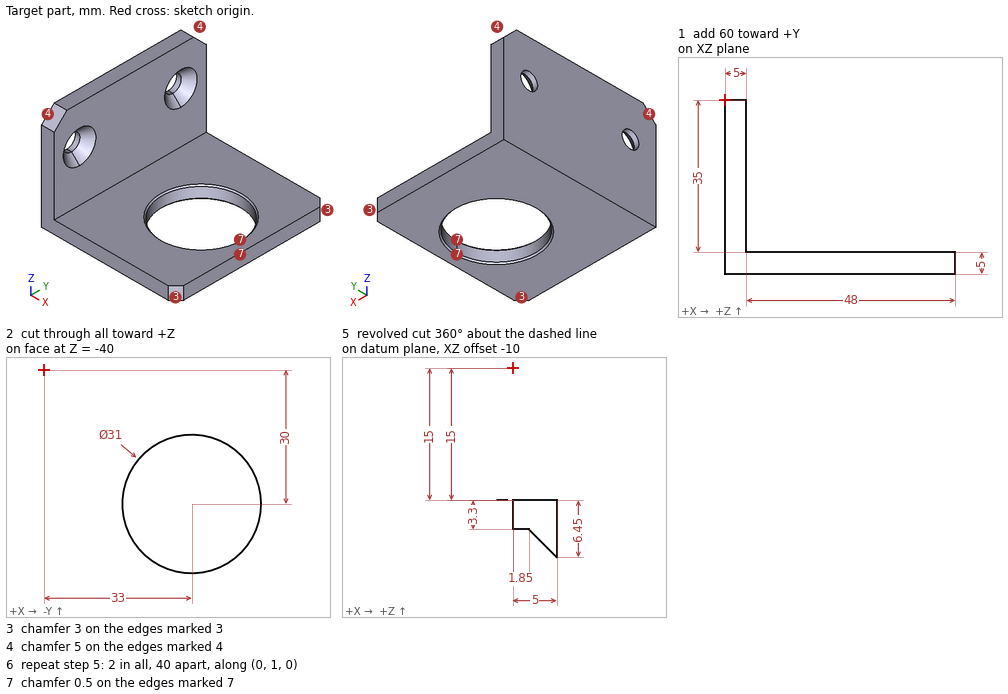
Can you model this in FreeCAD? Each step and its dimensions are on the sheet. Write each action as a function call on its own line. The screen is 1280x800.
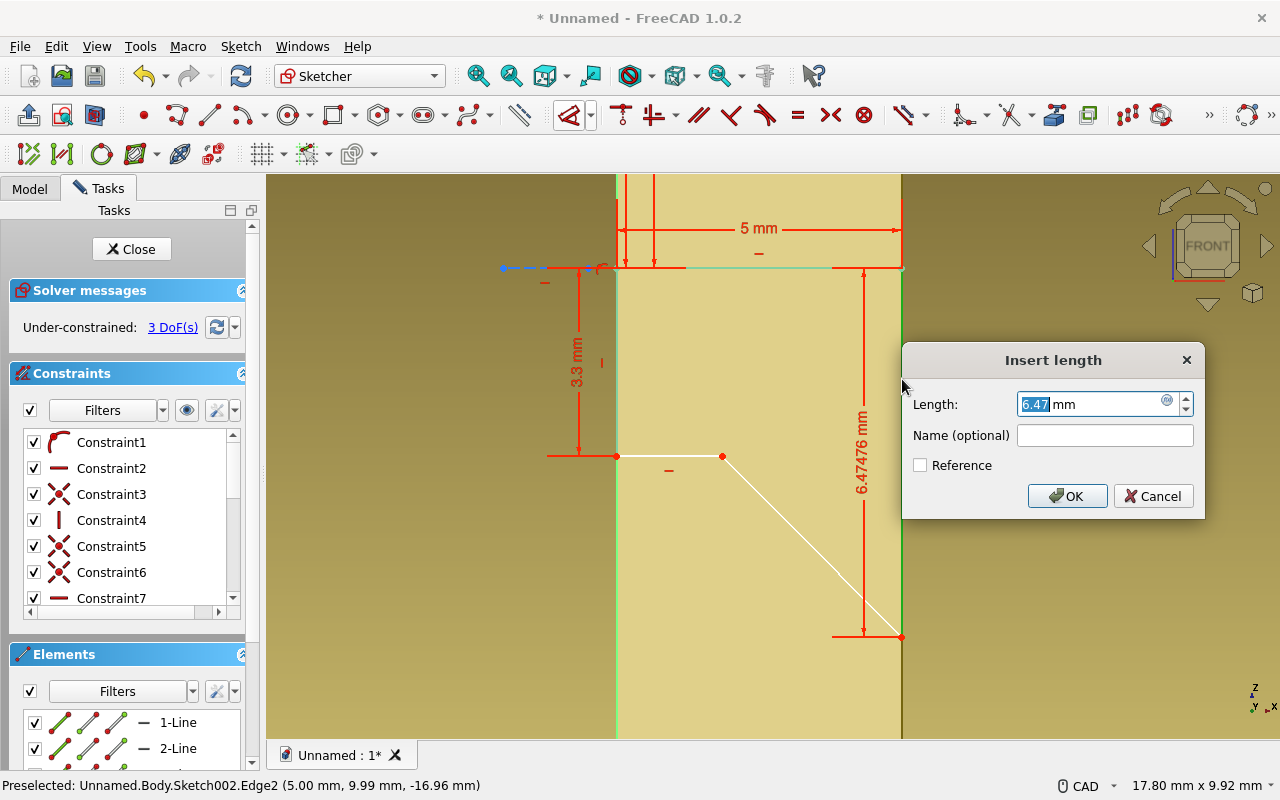
text(6.45)
key(Return)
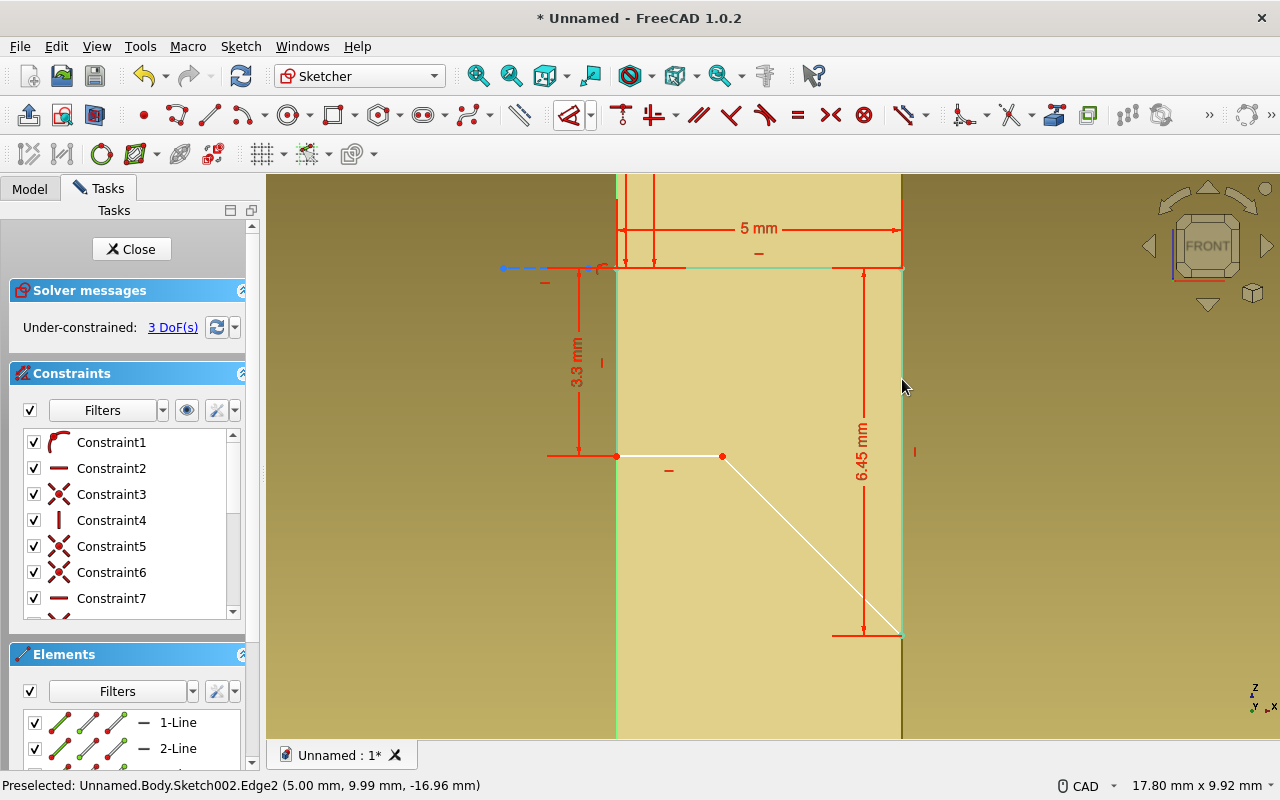
click(690, 456)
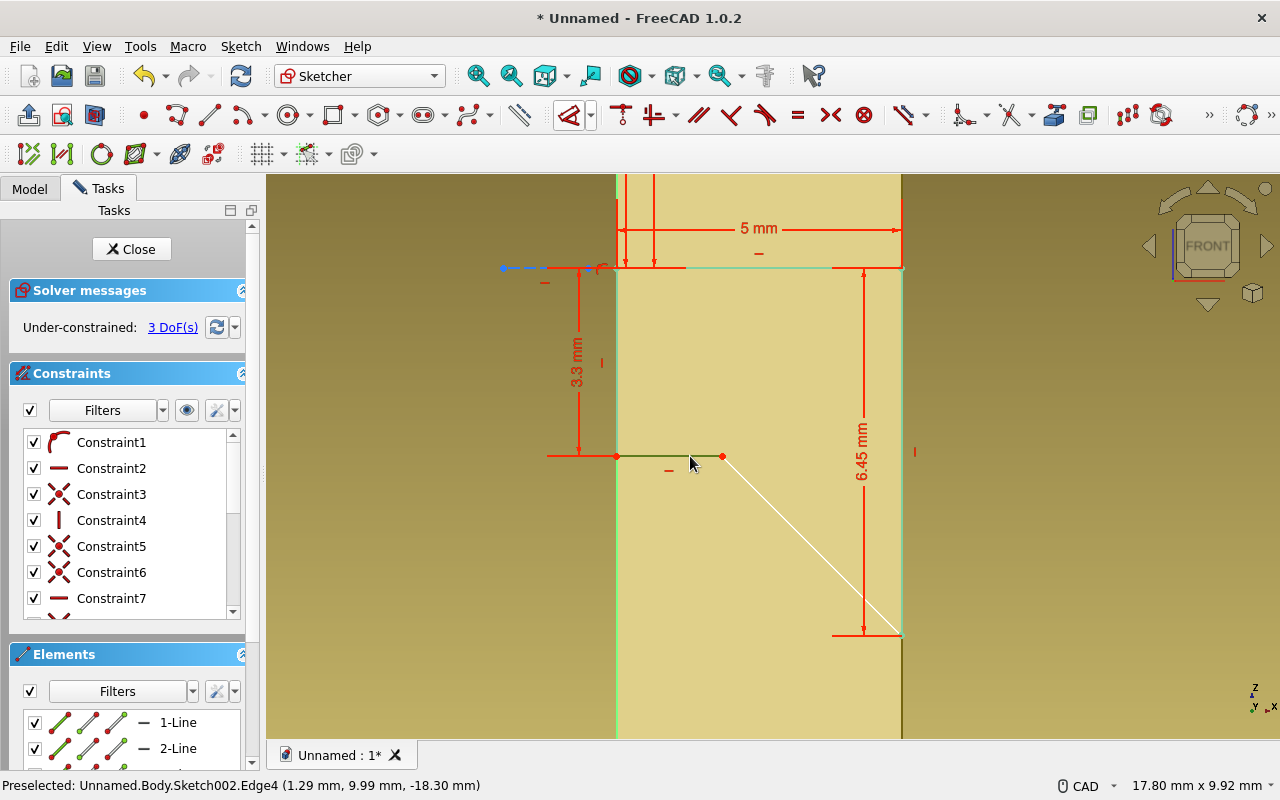
key(l)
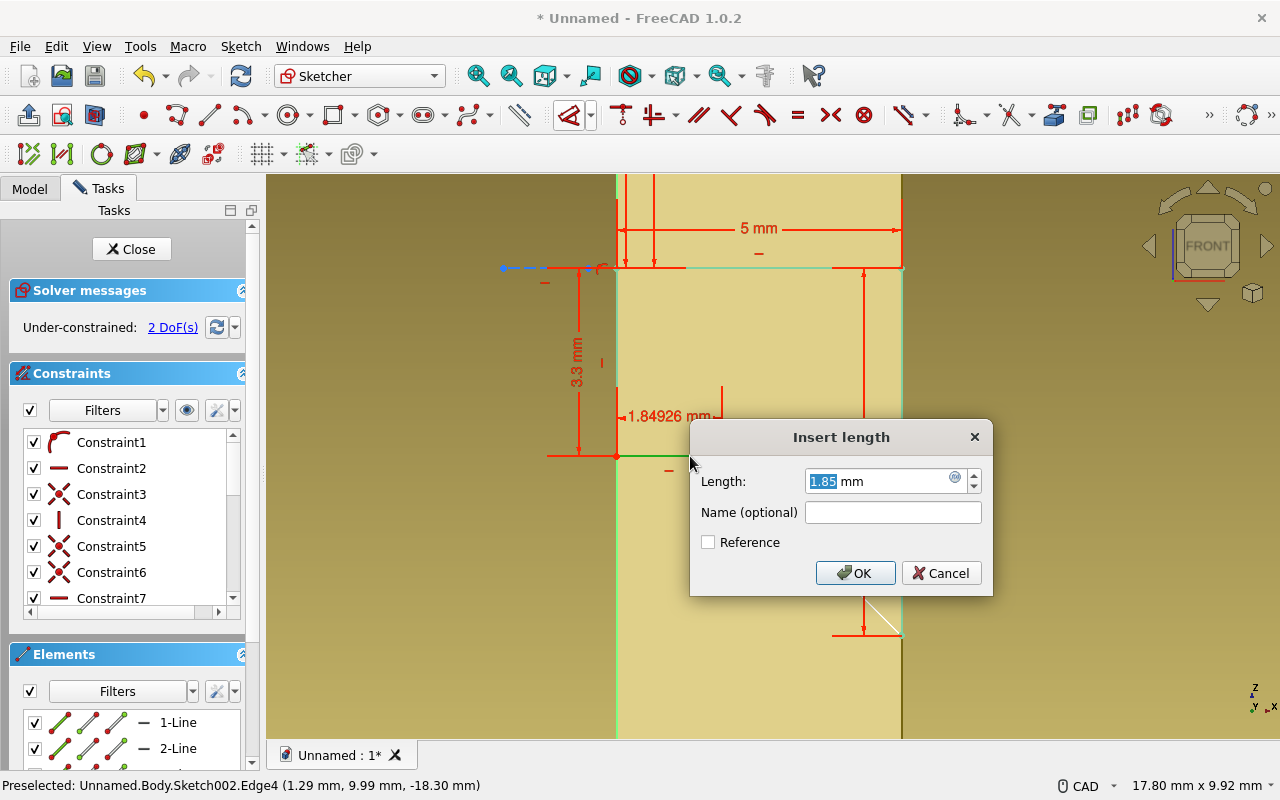
text(1.85)
key(Return)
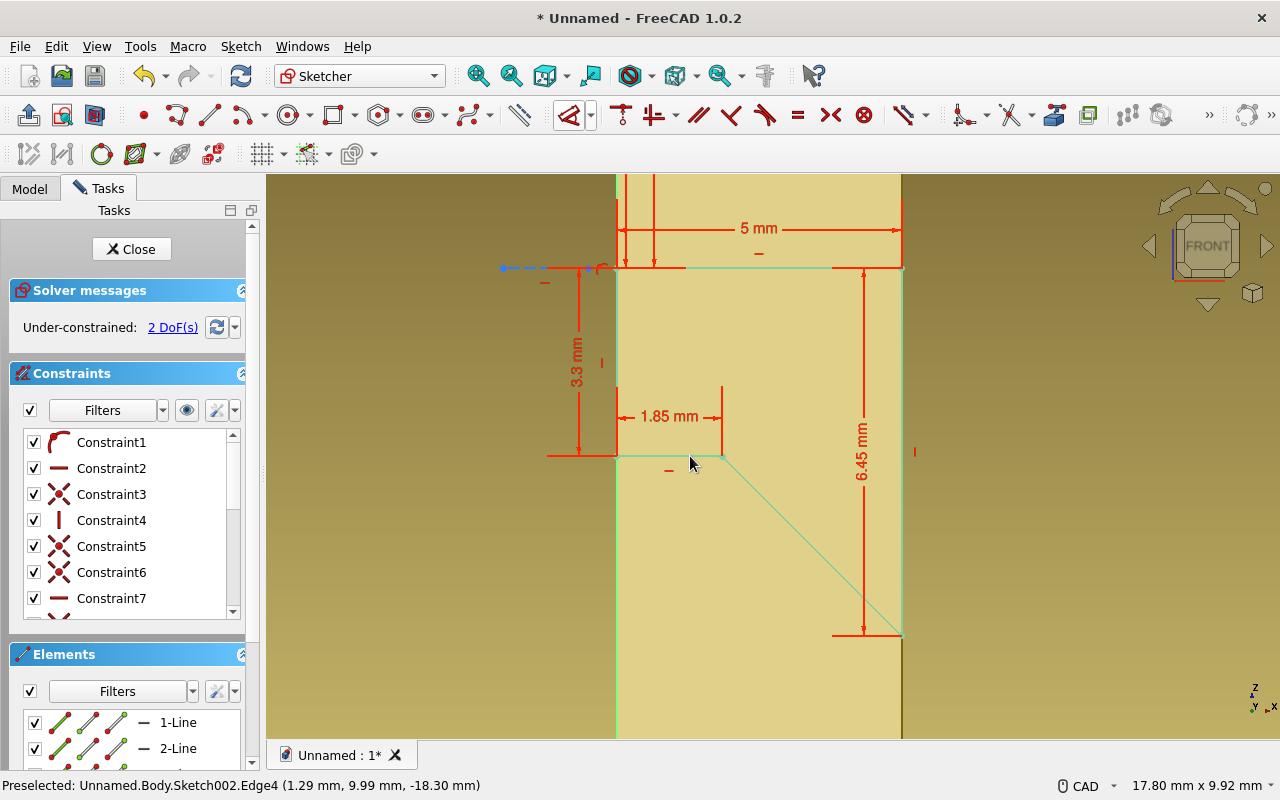
click(132, 249)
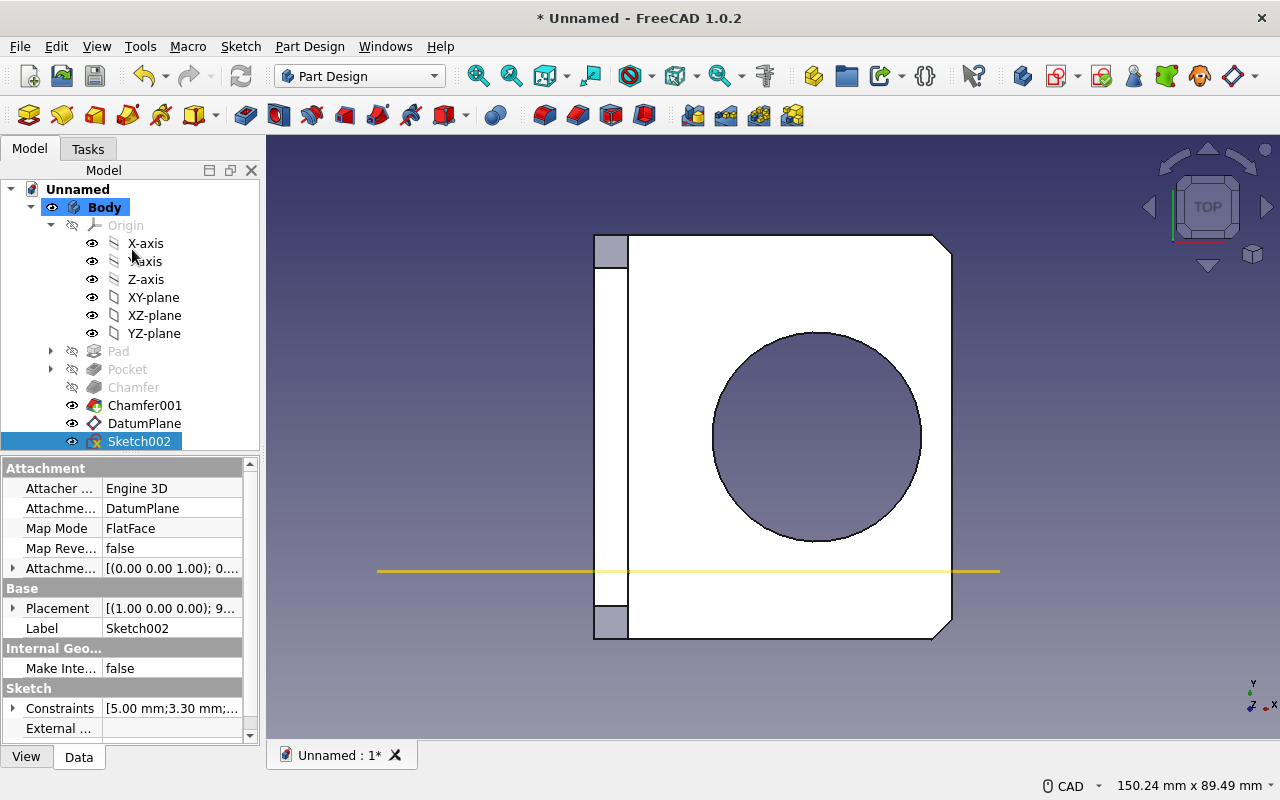
click(312, 116)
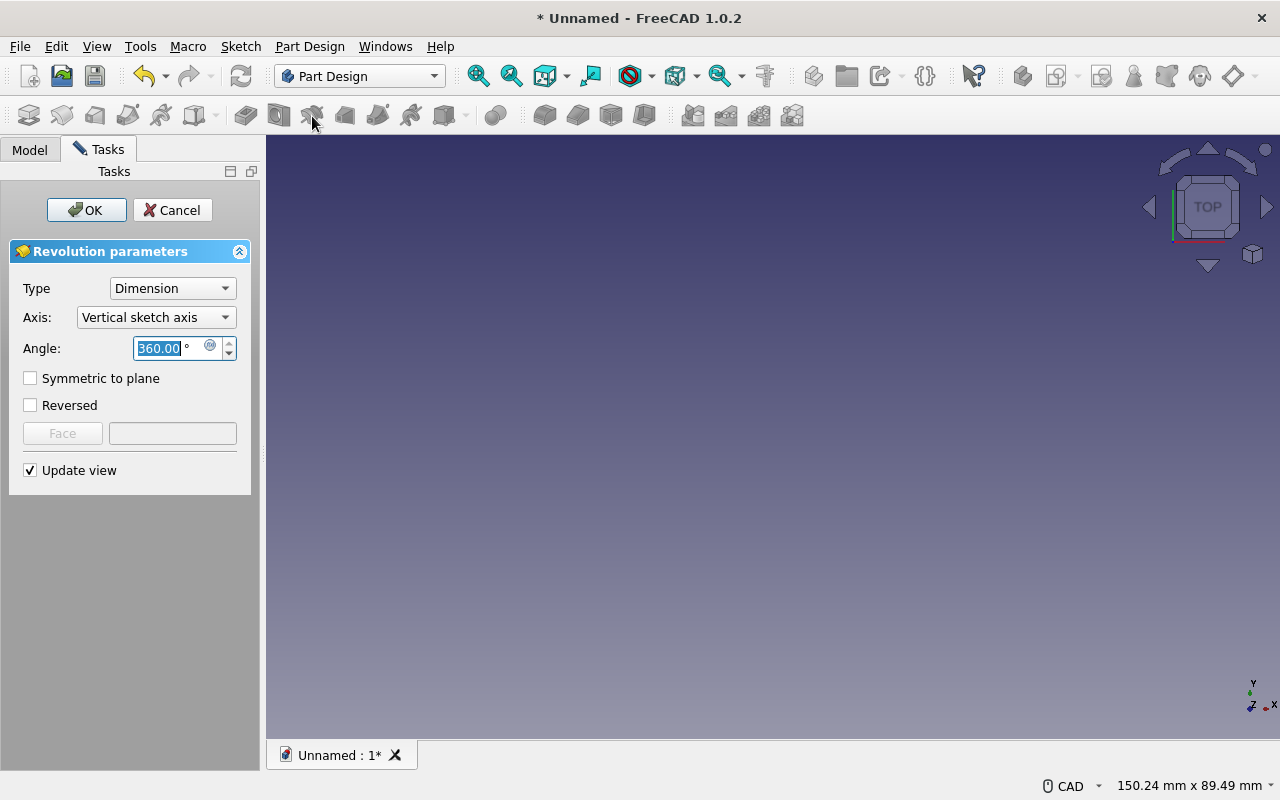
click(157, 318)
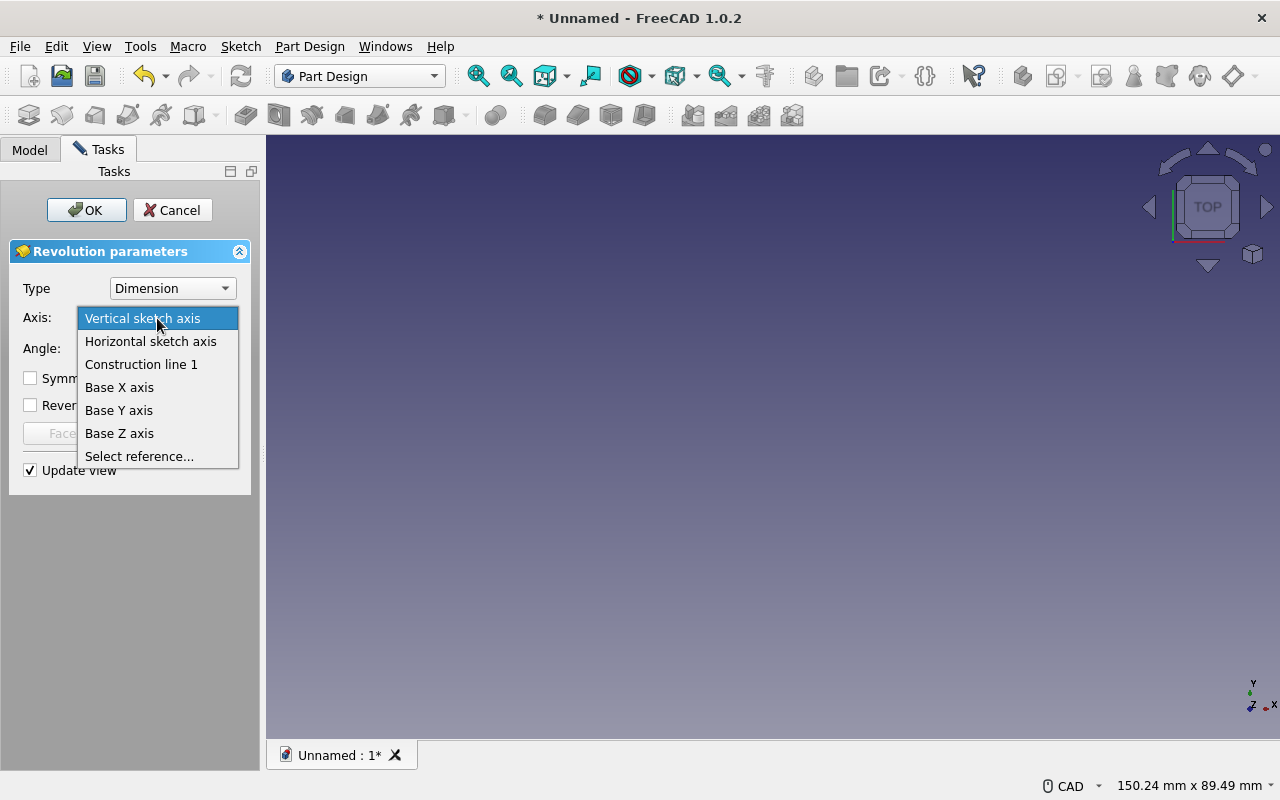
click(156, 364)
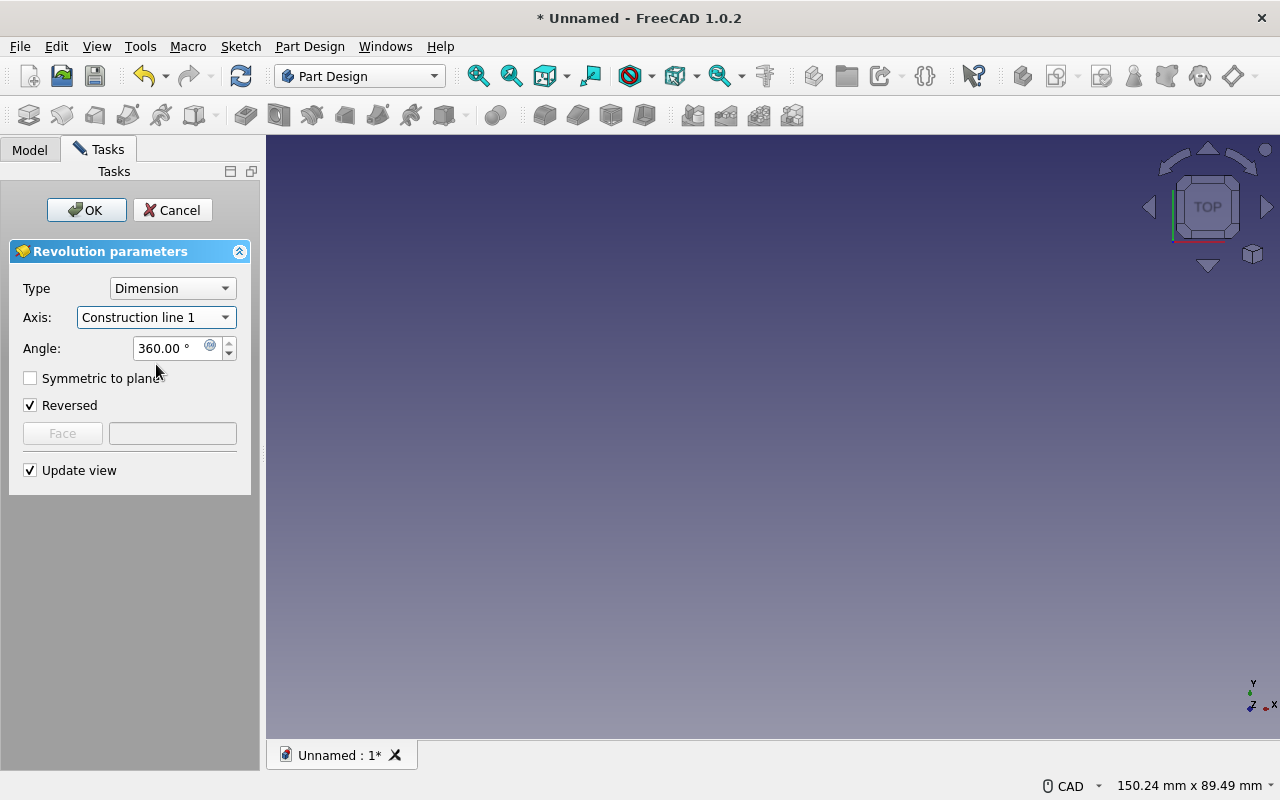
click(87, 210)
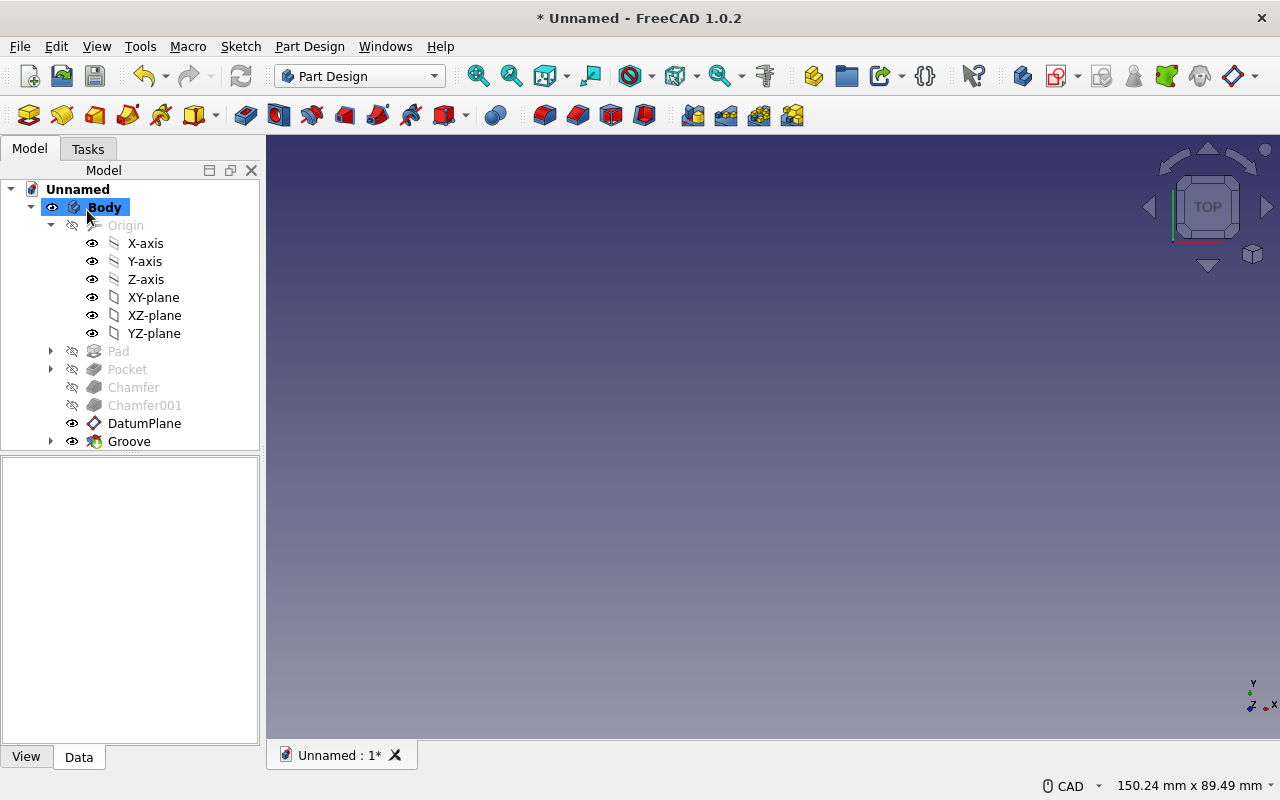
click(117, 423)
key(space)